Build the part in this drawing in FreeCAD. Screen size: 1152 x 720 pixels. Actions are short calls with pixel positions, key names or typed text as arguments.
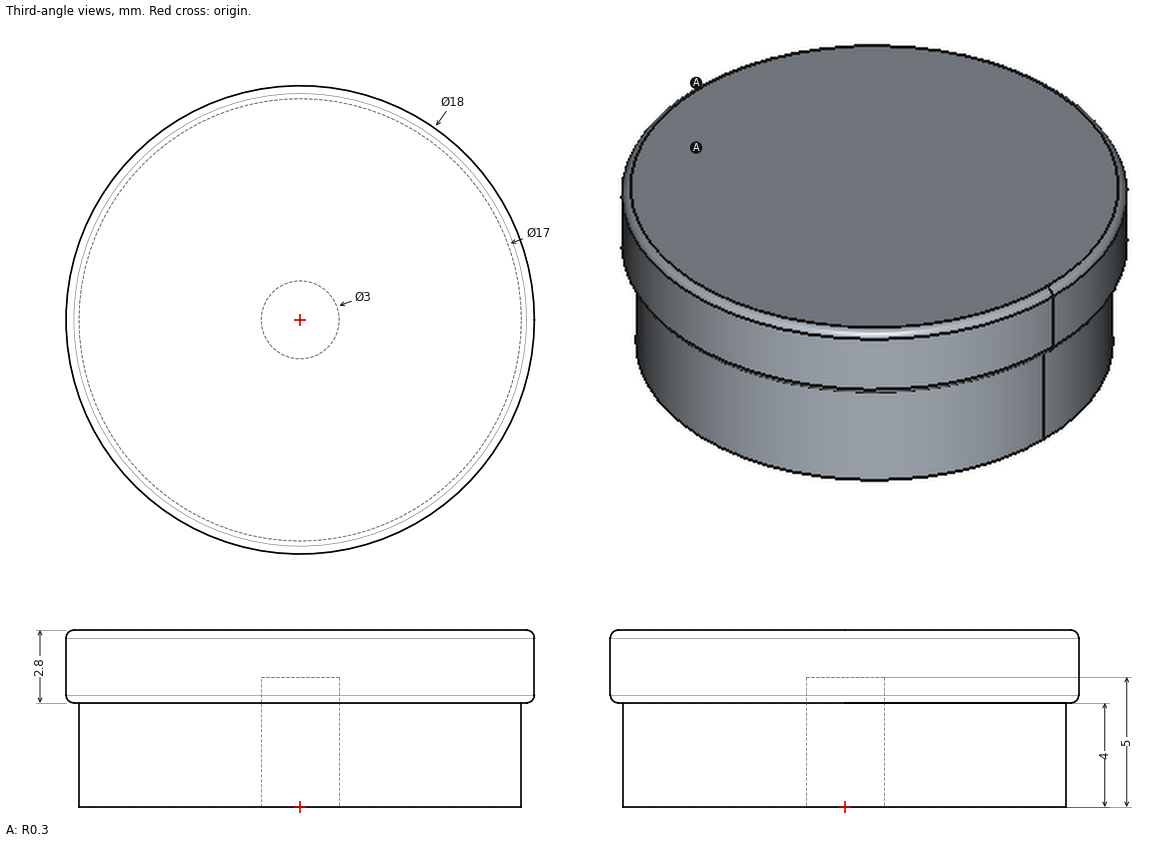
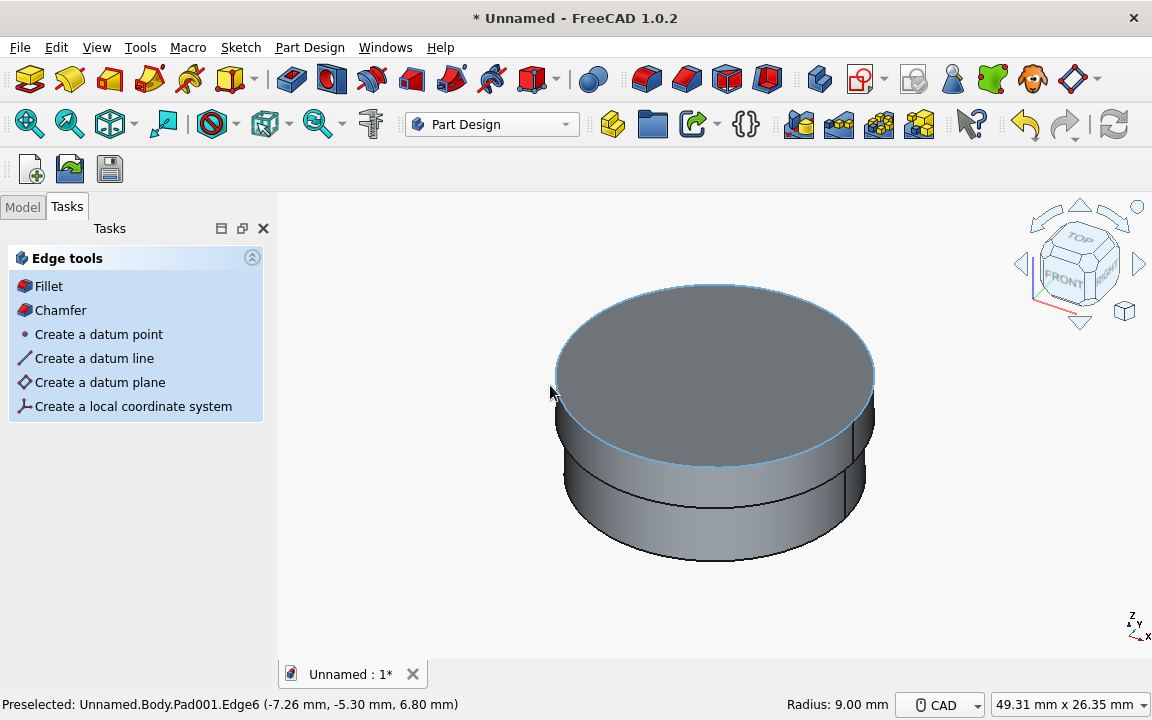
key(0)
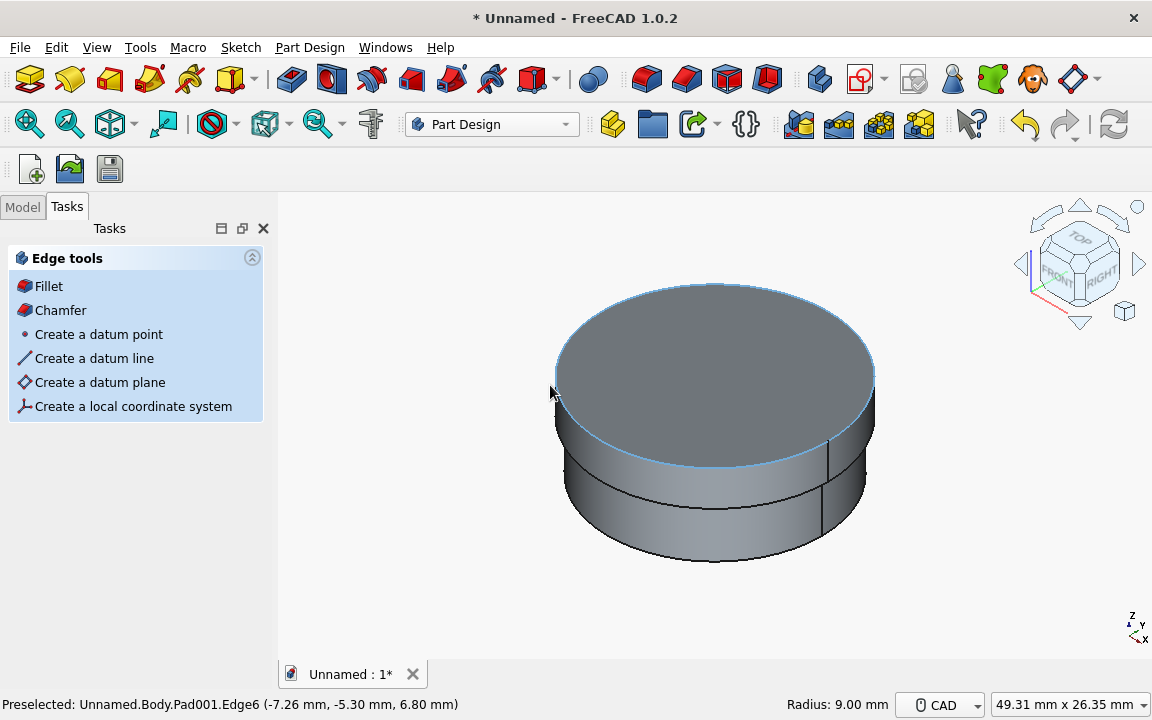
key(2)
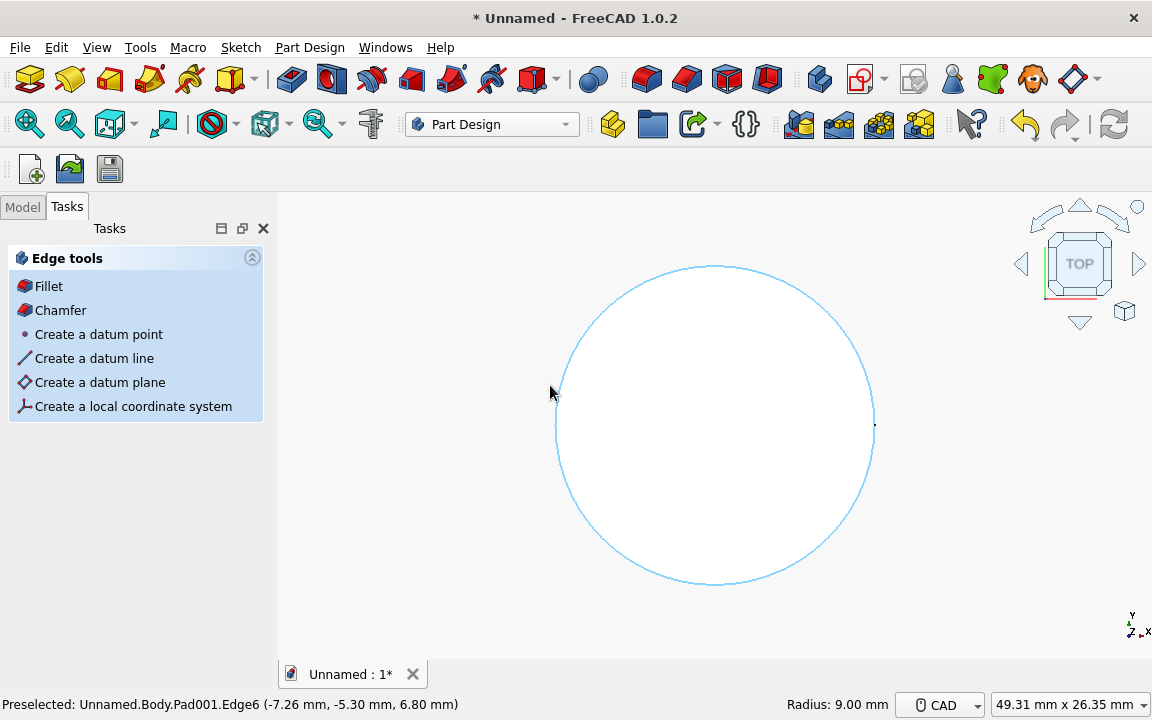
key(1)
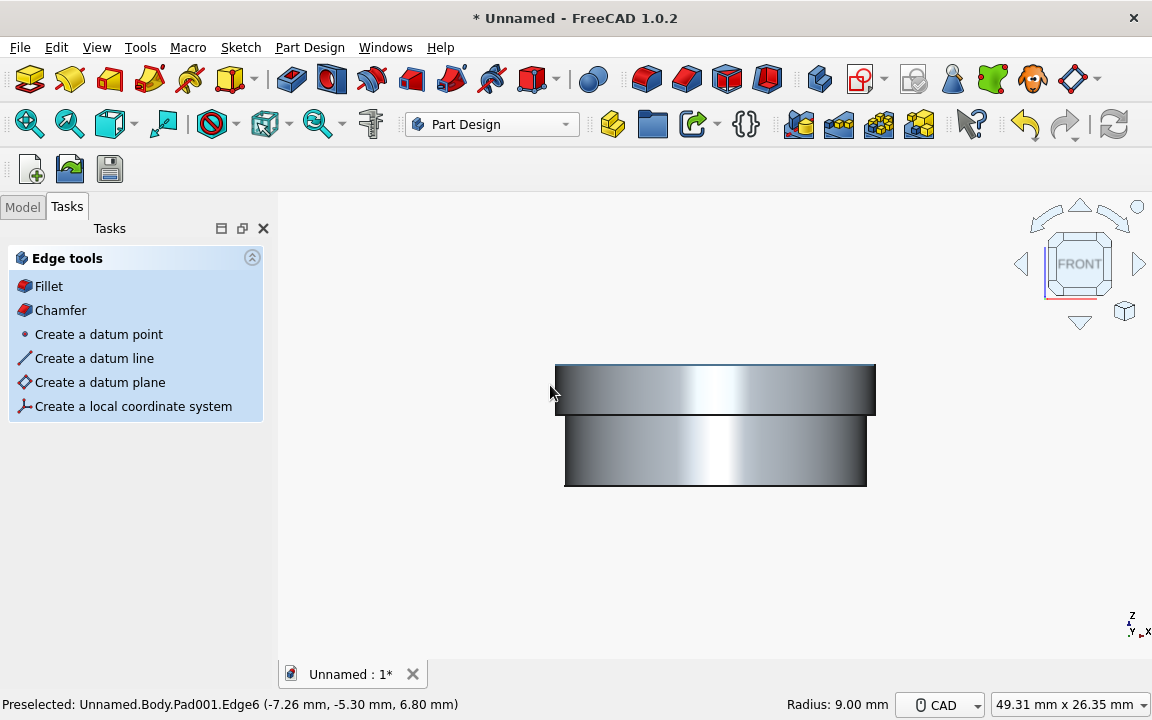
click(30, 124)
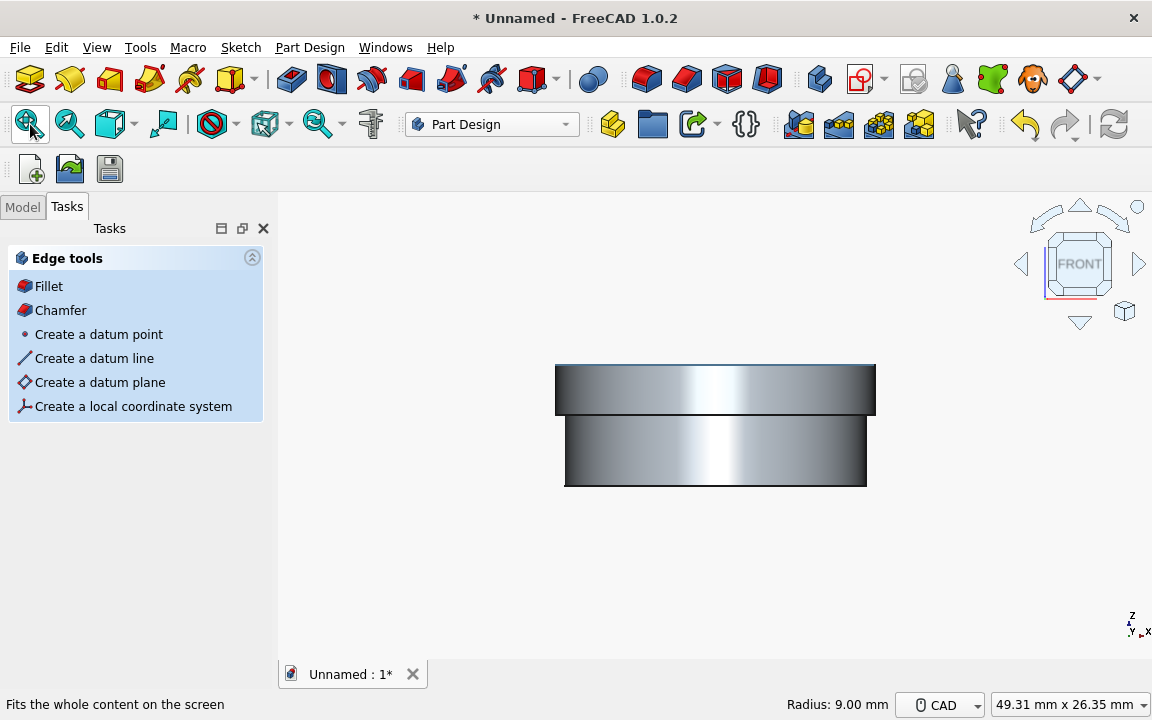
click(586, 414, ctrl)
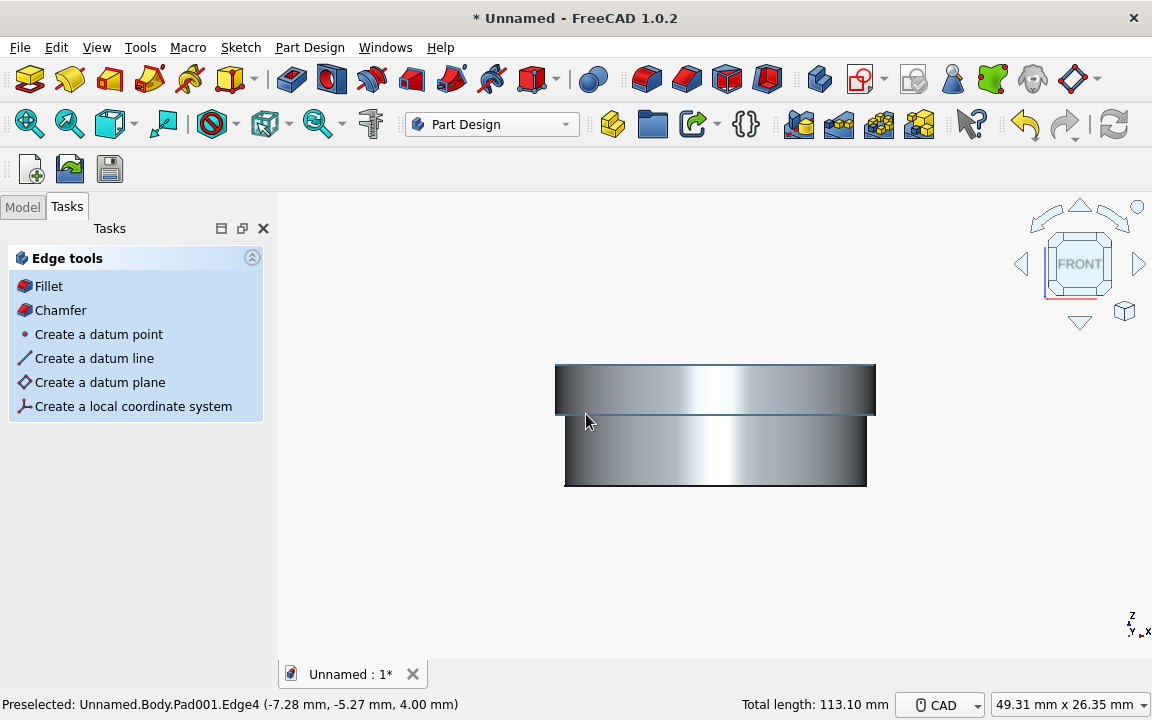
click(648, 80)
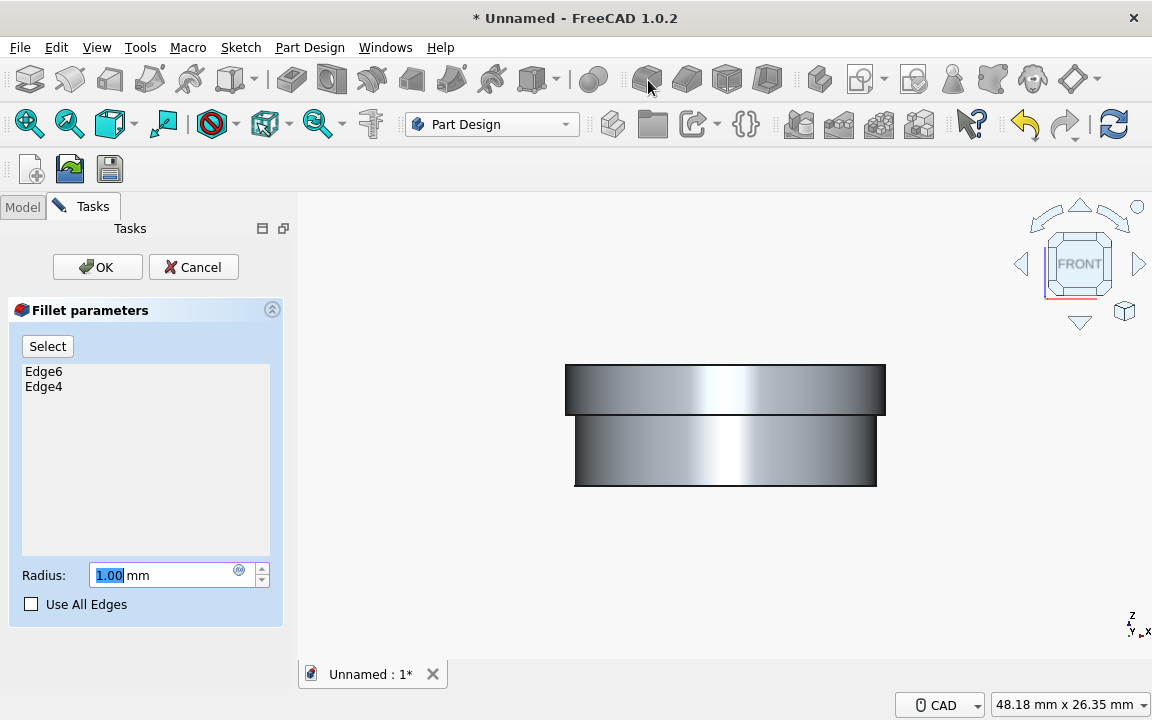
text(0.3)
key(Tab)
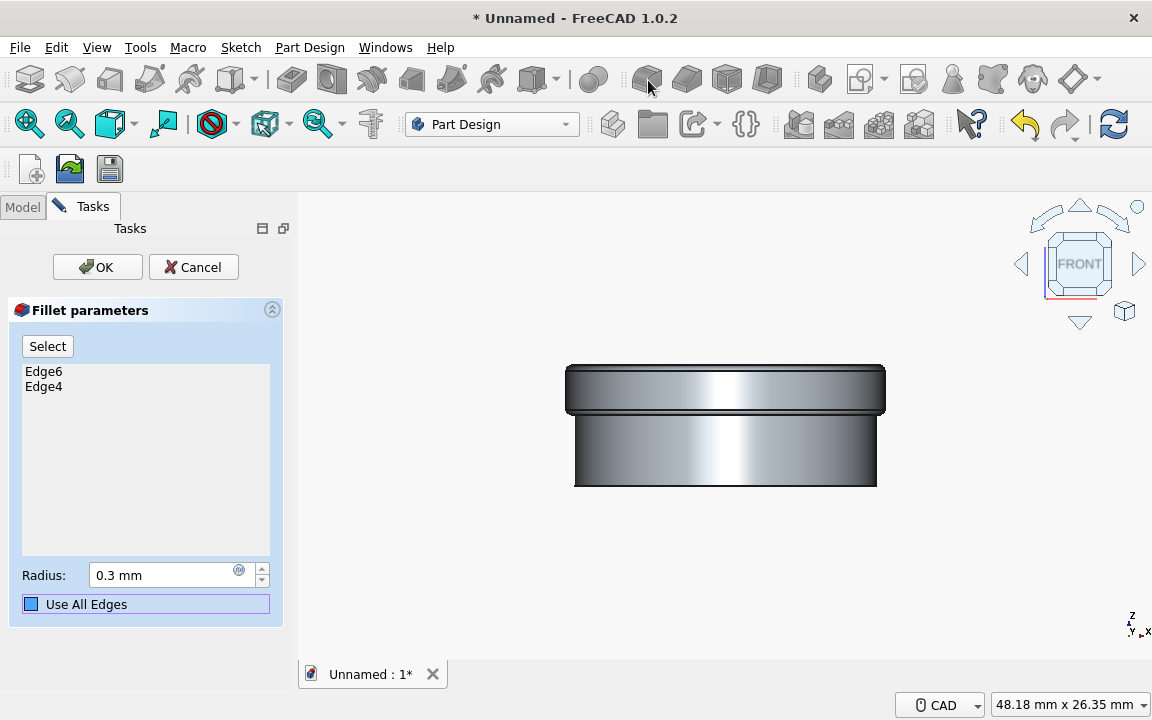
click(98, 267)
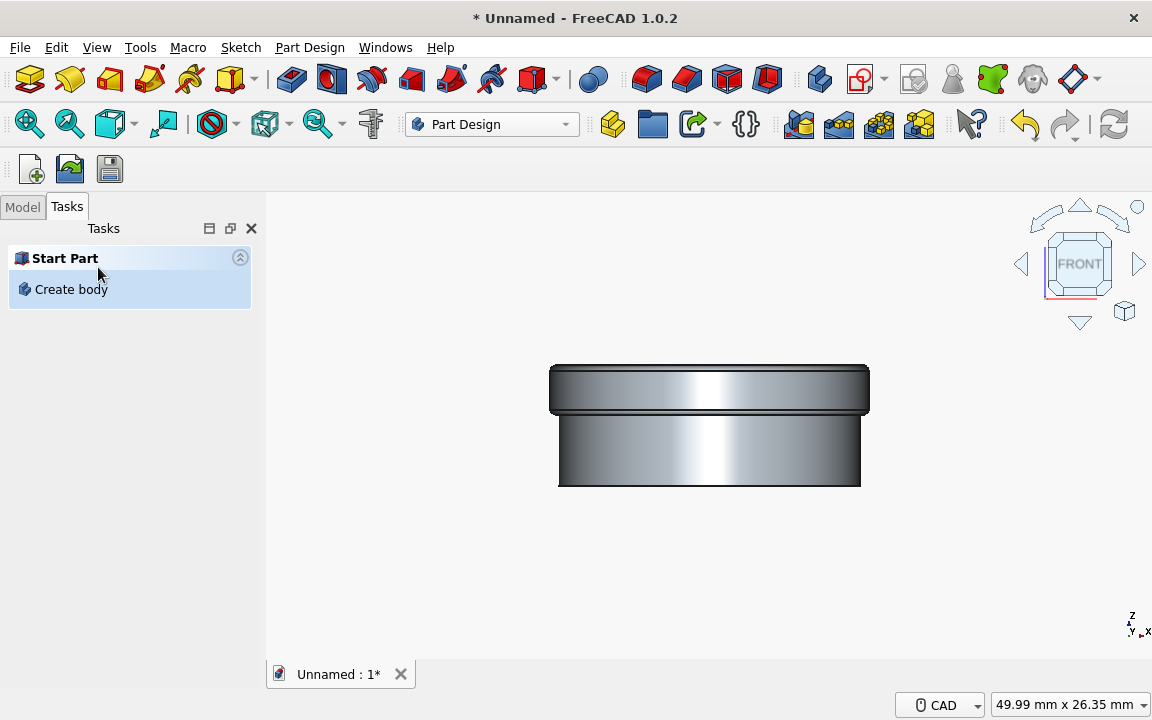
click(30, 124)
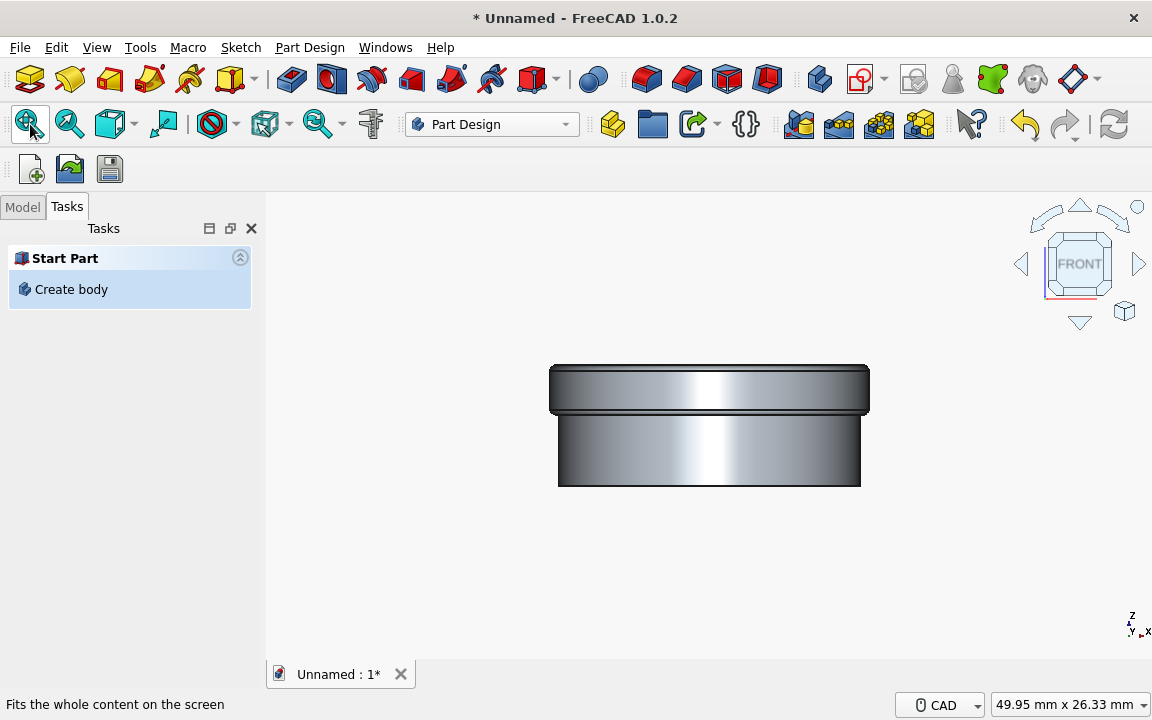
key(5)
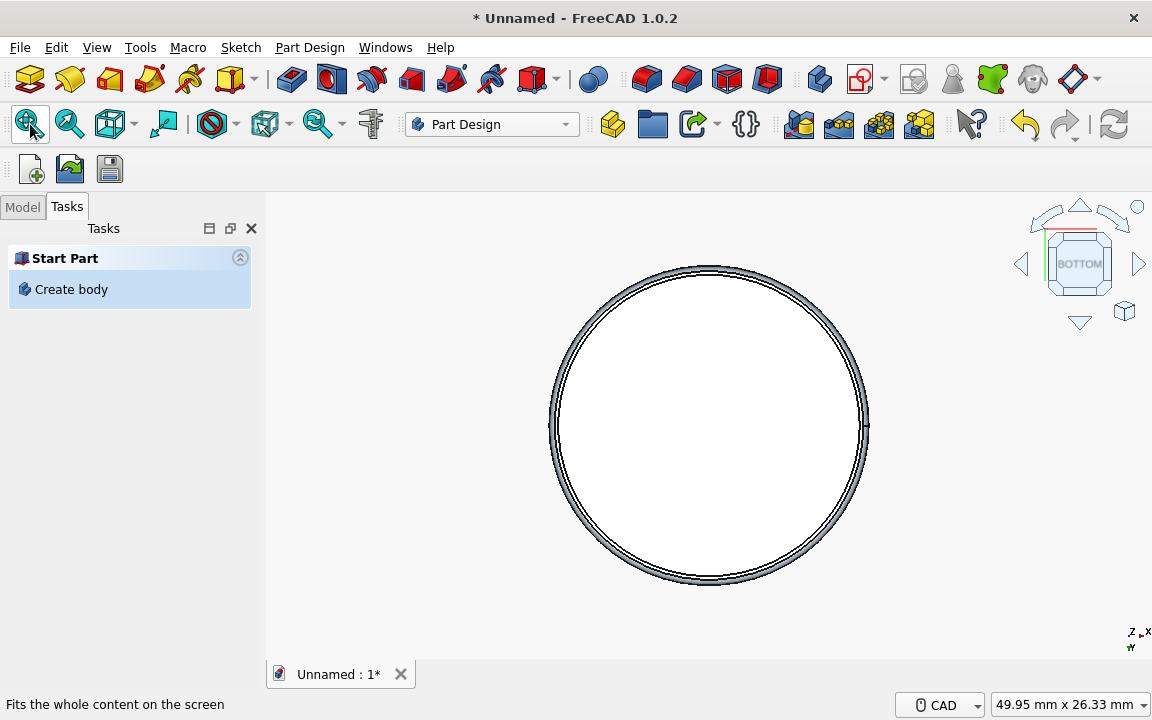
click(709, 424)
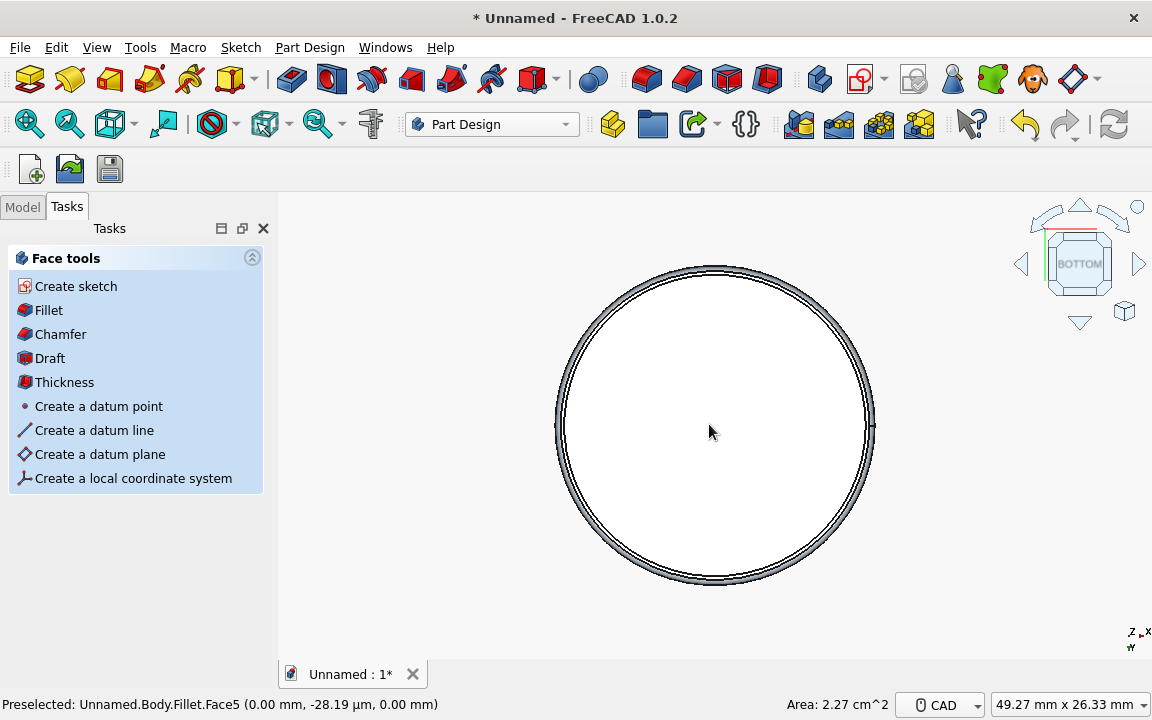
click(860, 80)